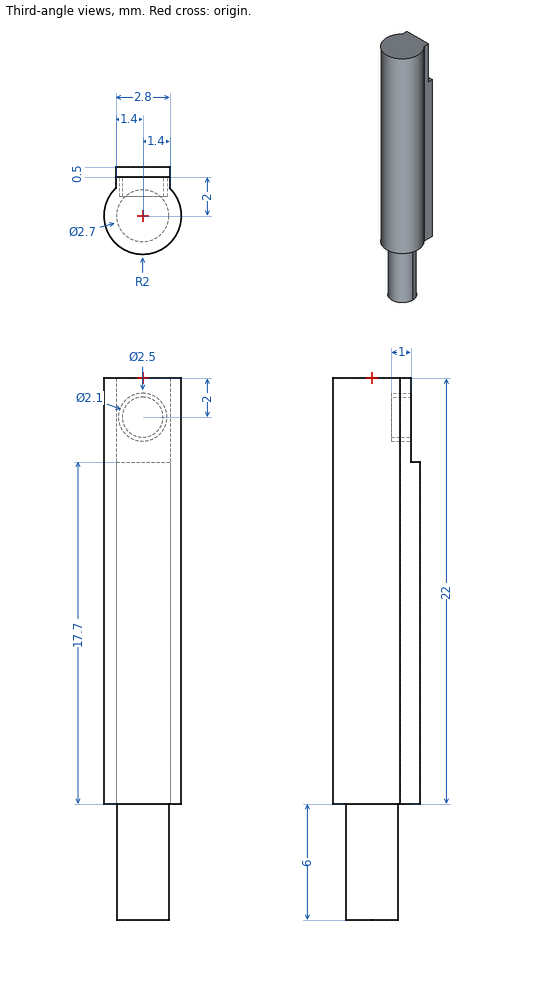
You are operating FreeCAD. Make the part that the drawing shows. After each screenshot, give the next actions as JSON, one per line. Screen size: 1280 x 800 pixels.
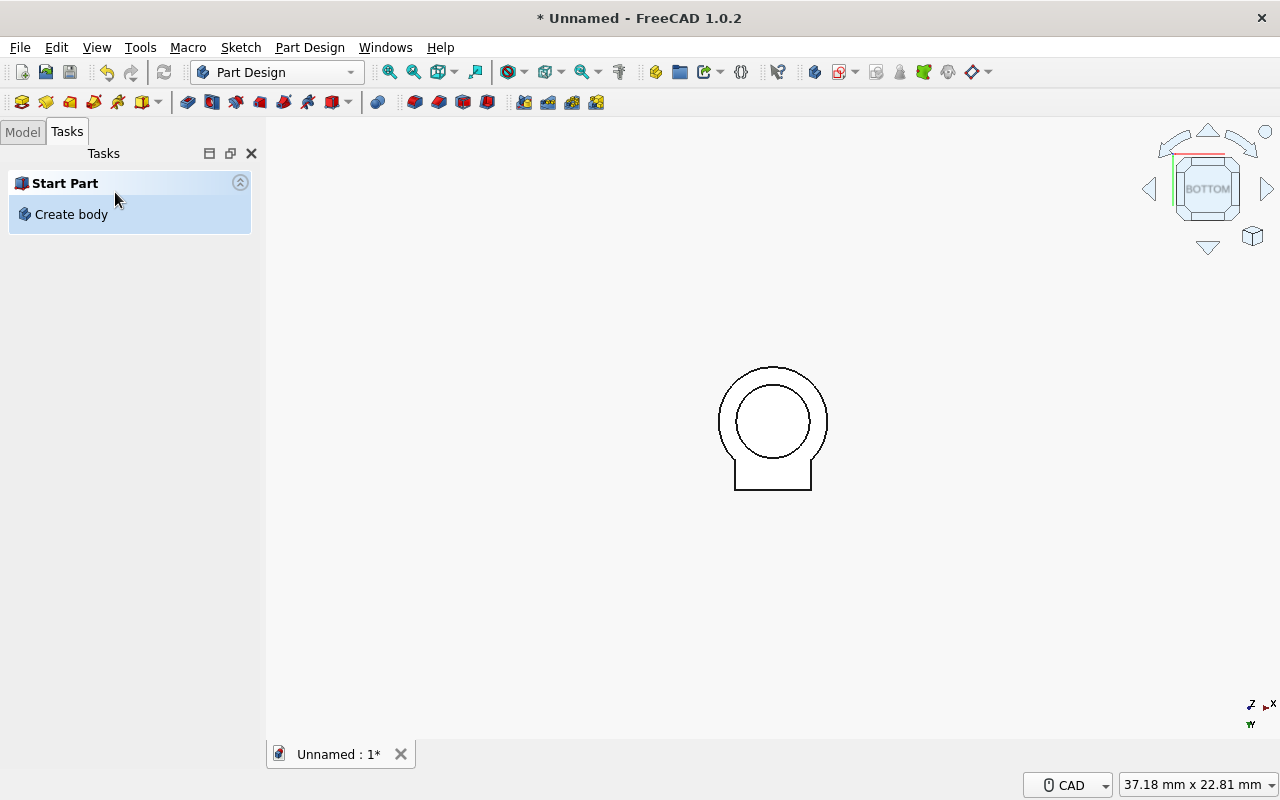
{"action": "key", "text": "0"}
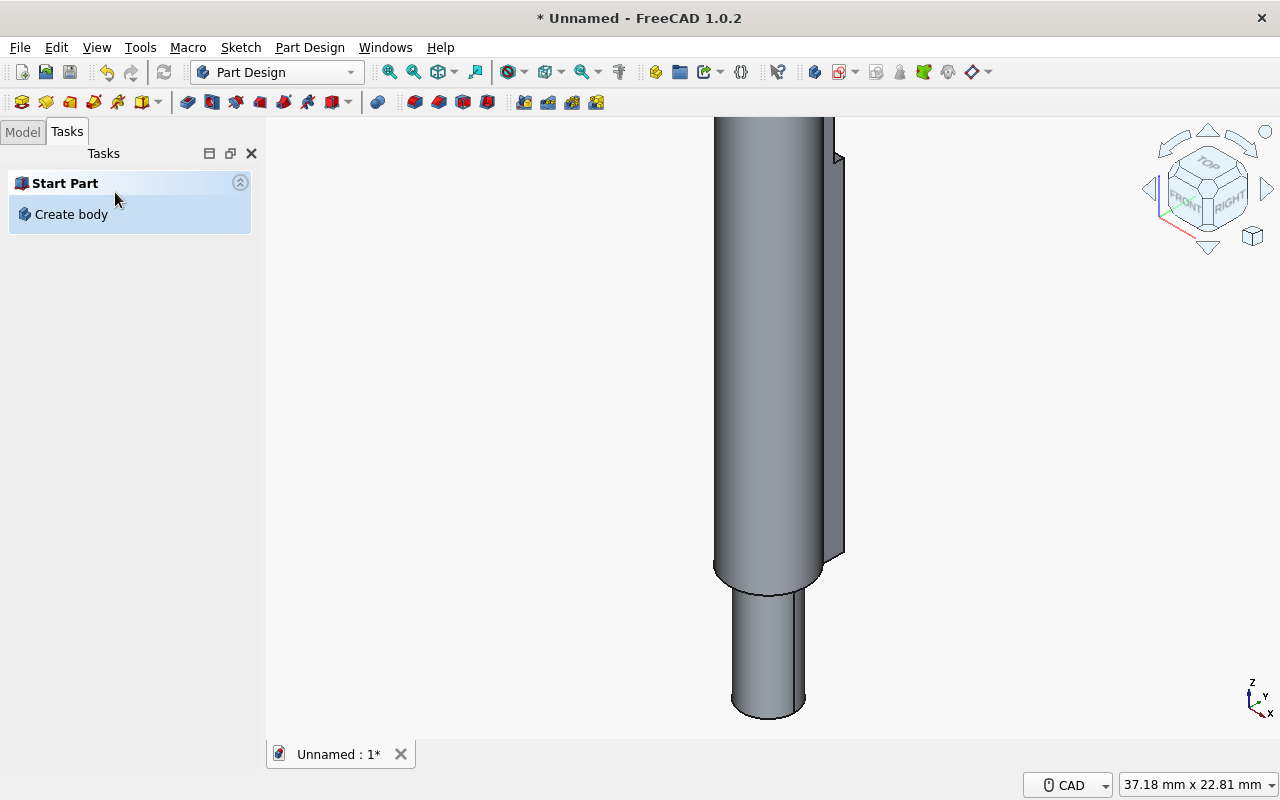
{"action": "left_click", "coordinate": [390, 72]}